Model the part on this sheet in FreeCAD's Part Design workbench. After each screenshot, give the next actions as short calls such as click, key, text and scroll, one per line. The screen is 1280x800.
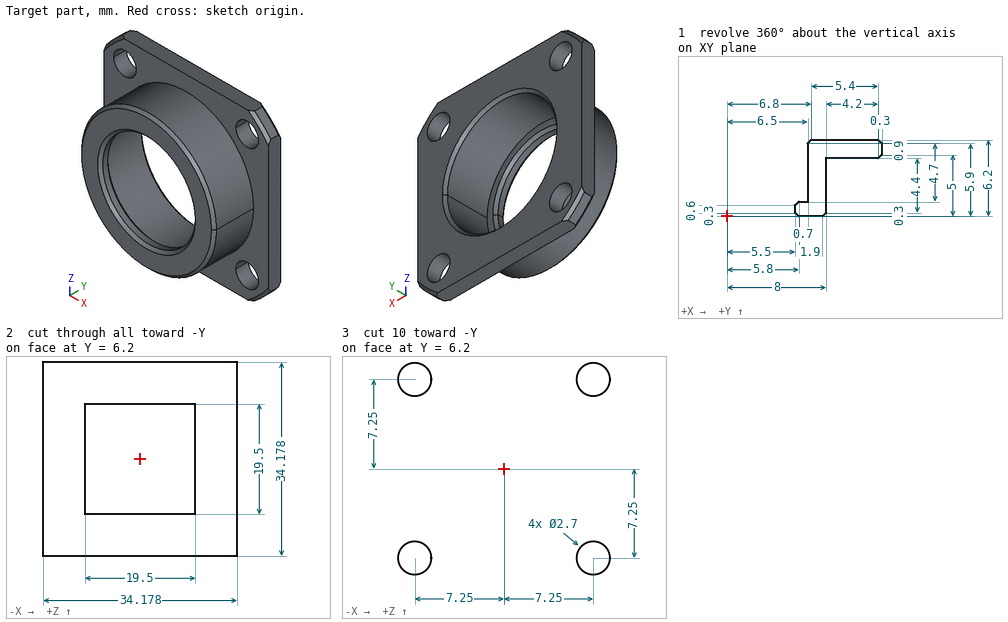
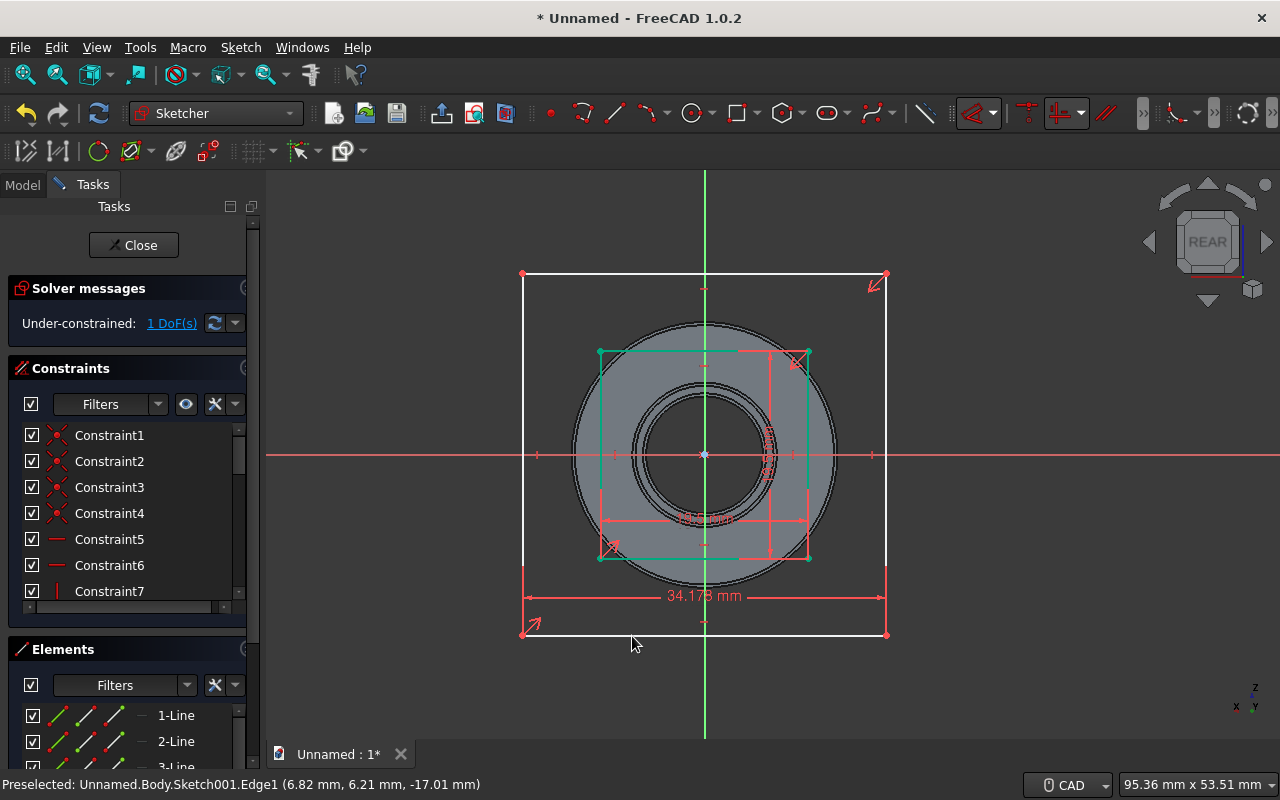
click(886, 527)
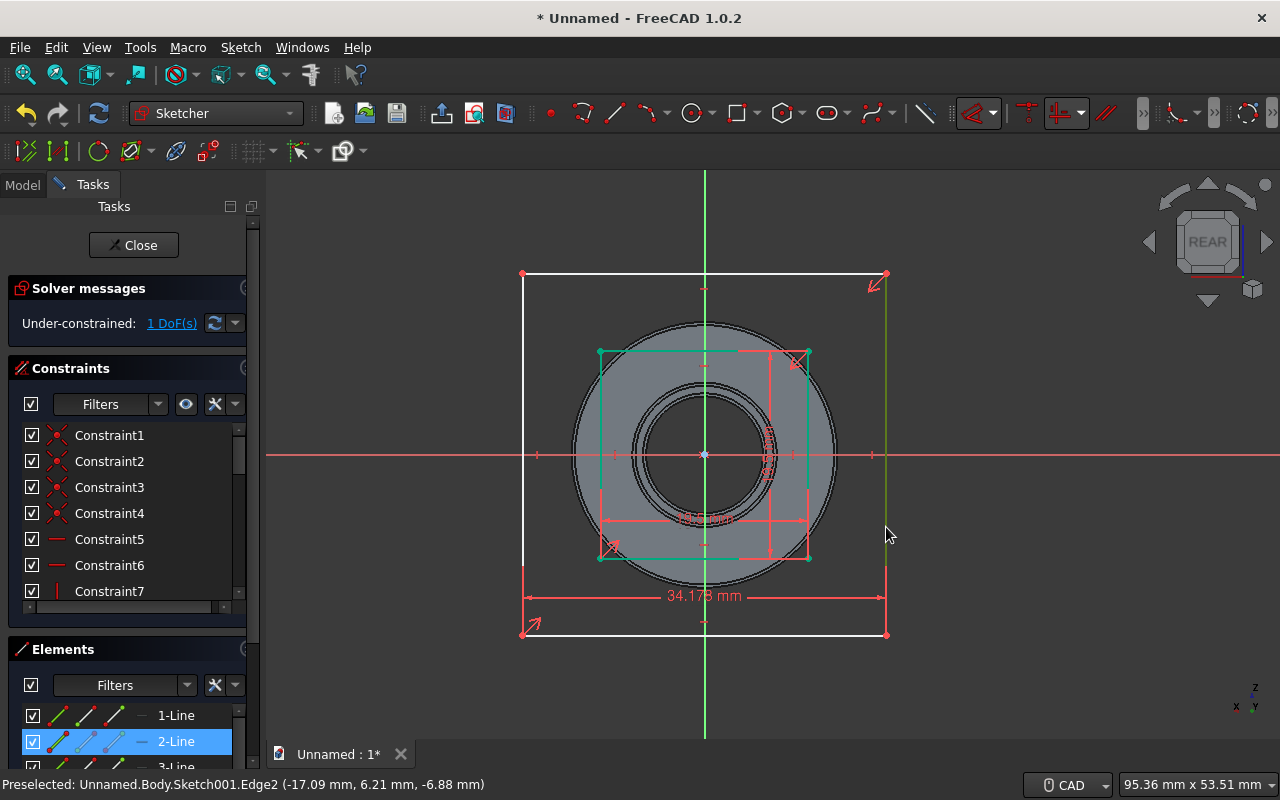
click(996, 114)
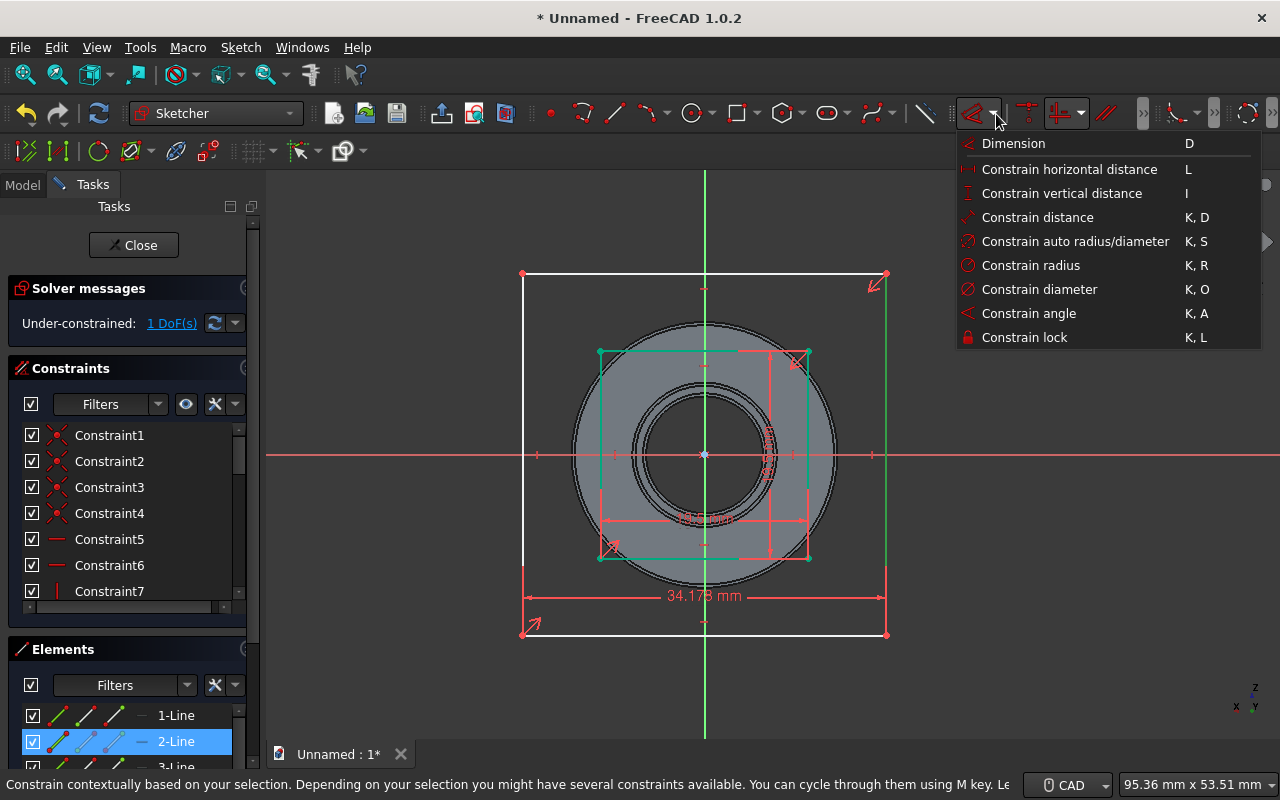
click(1109, 193)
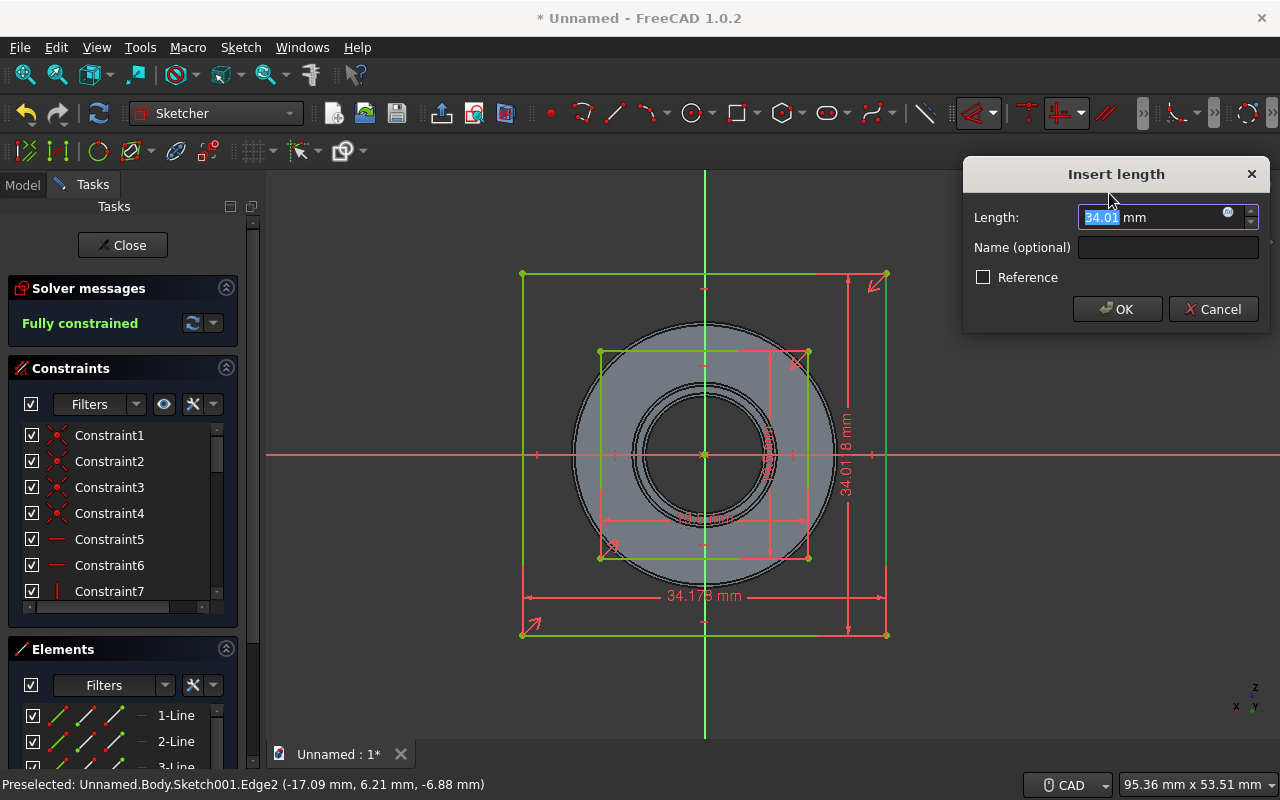
text(34.178)
key(Return)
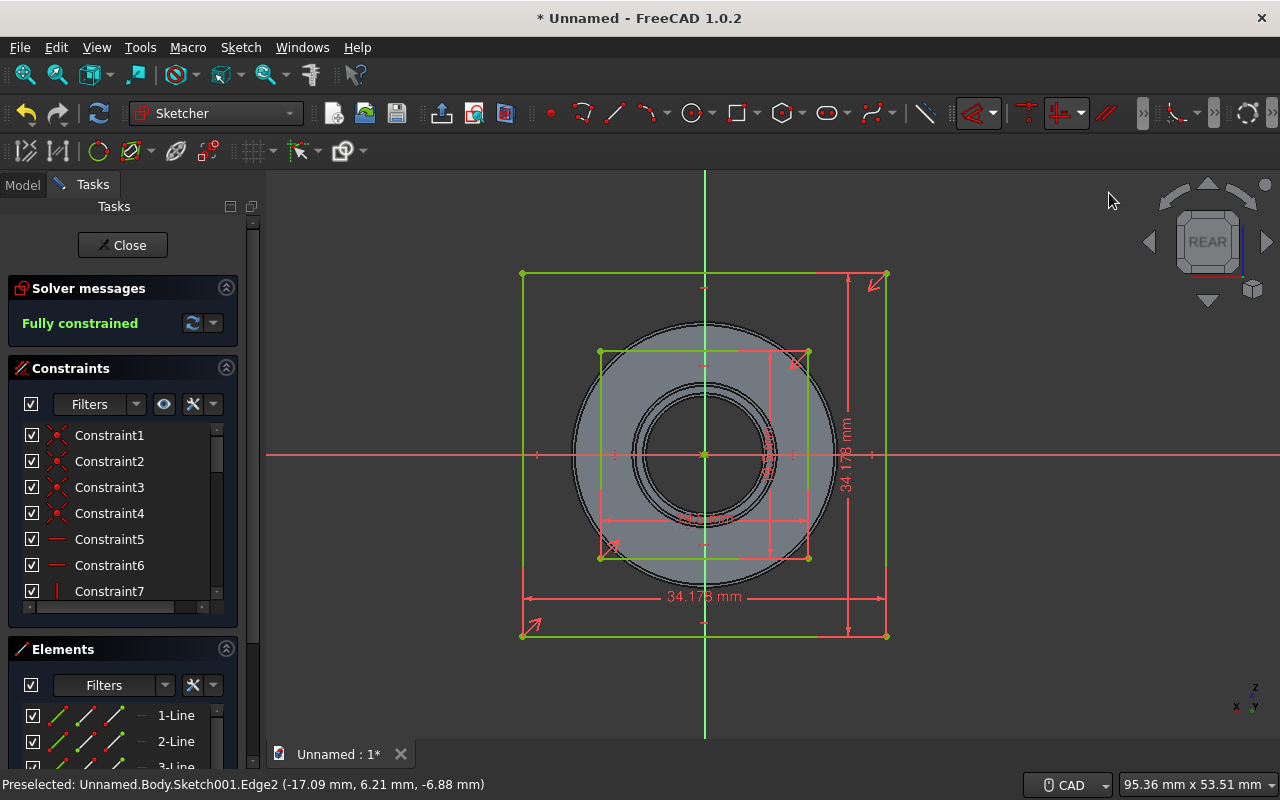
click(123, 245)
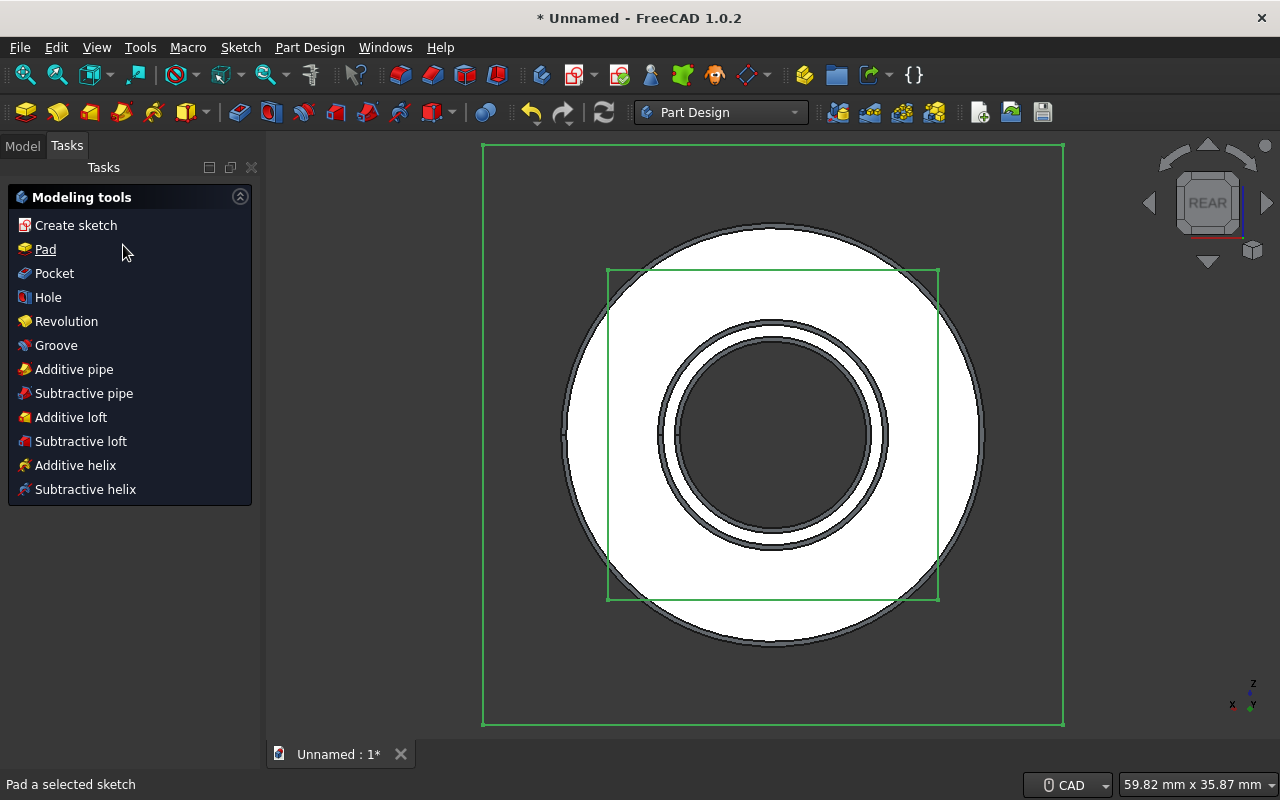
click(240, 112)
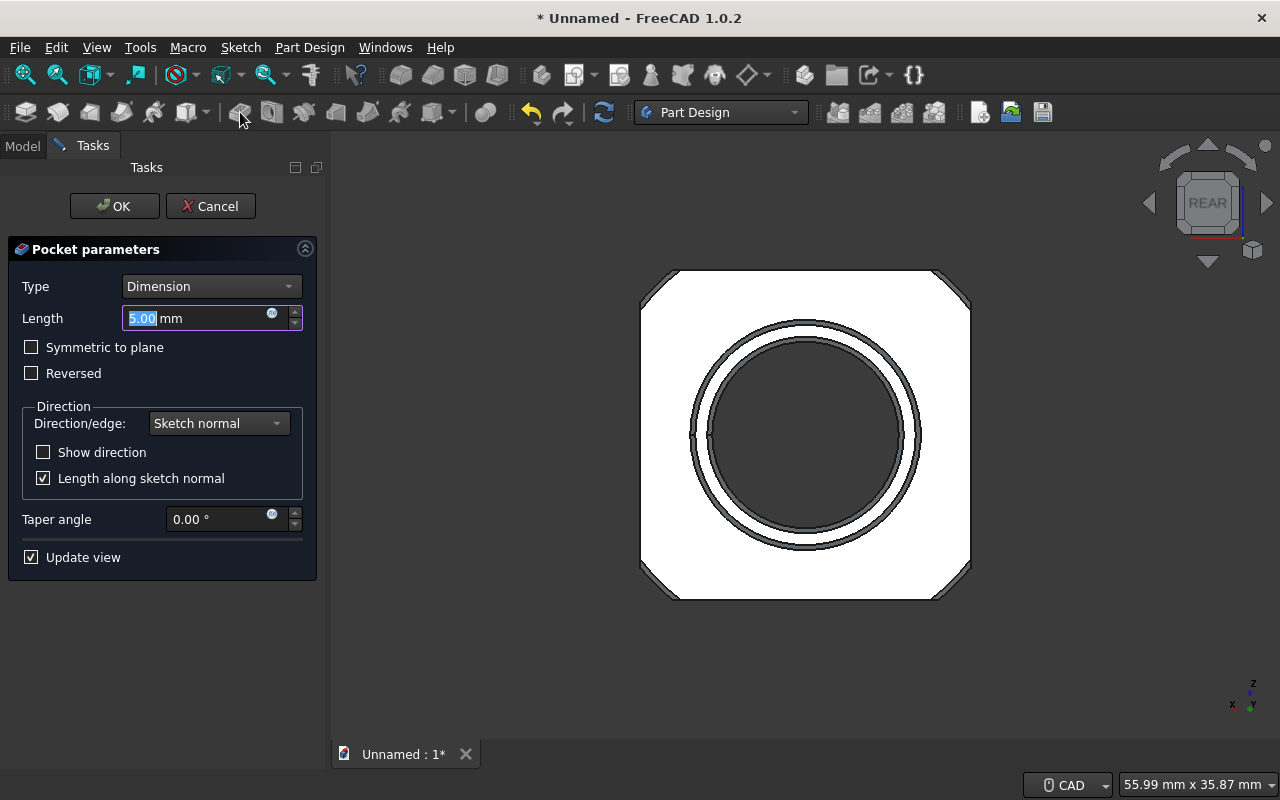
click(212, 286)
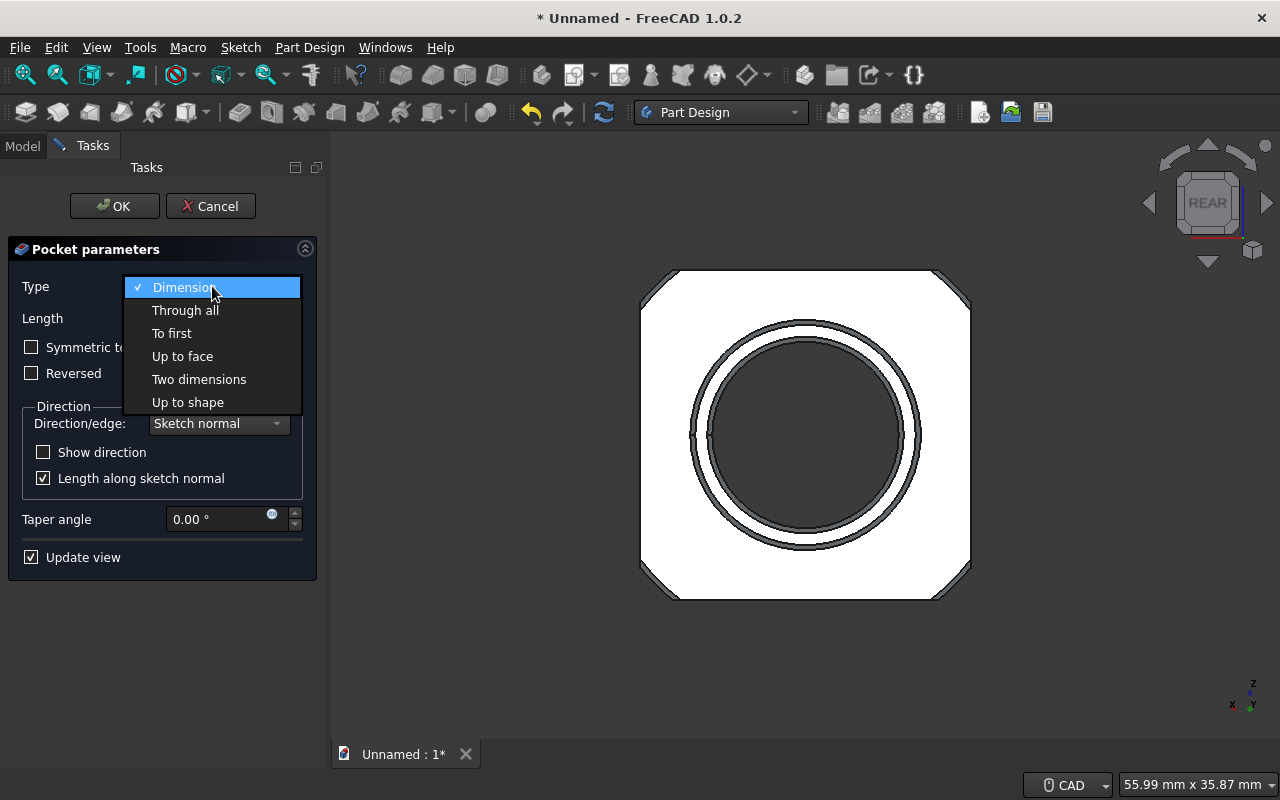
click(212, 310)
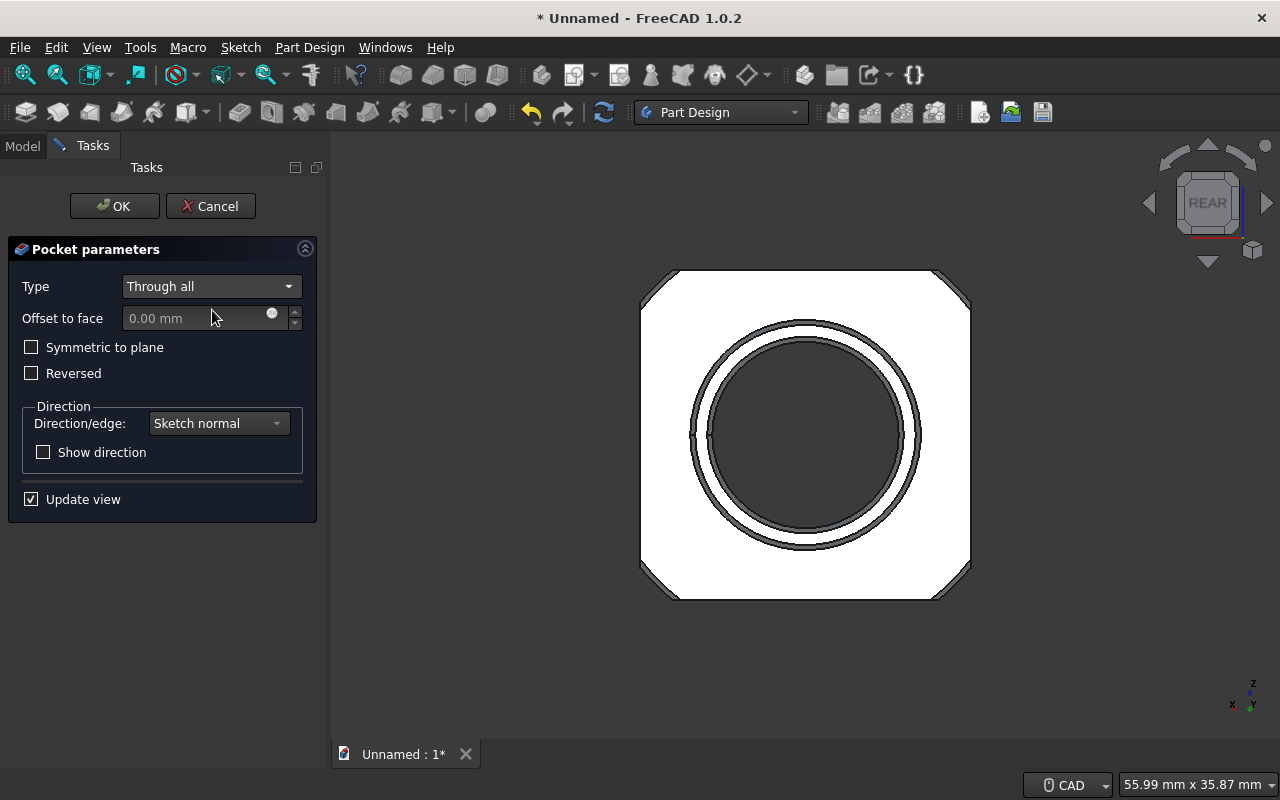
click(115, 206)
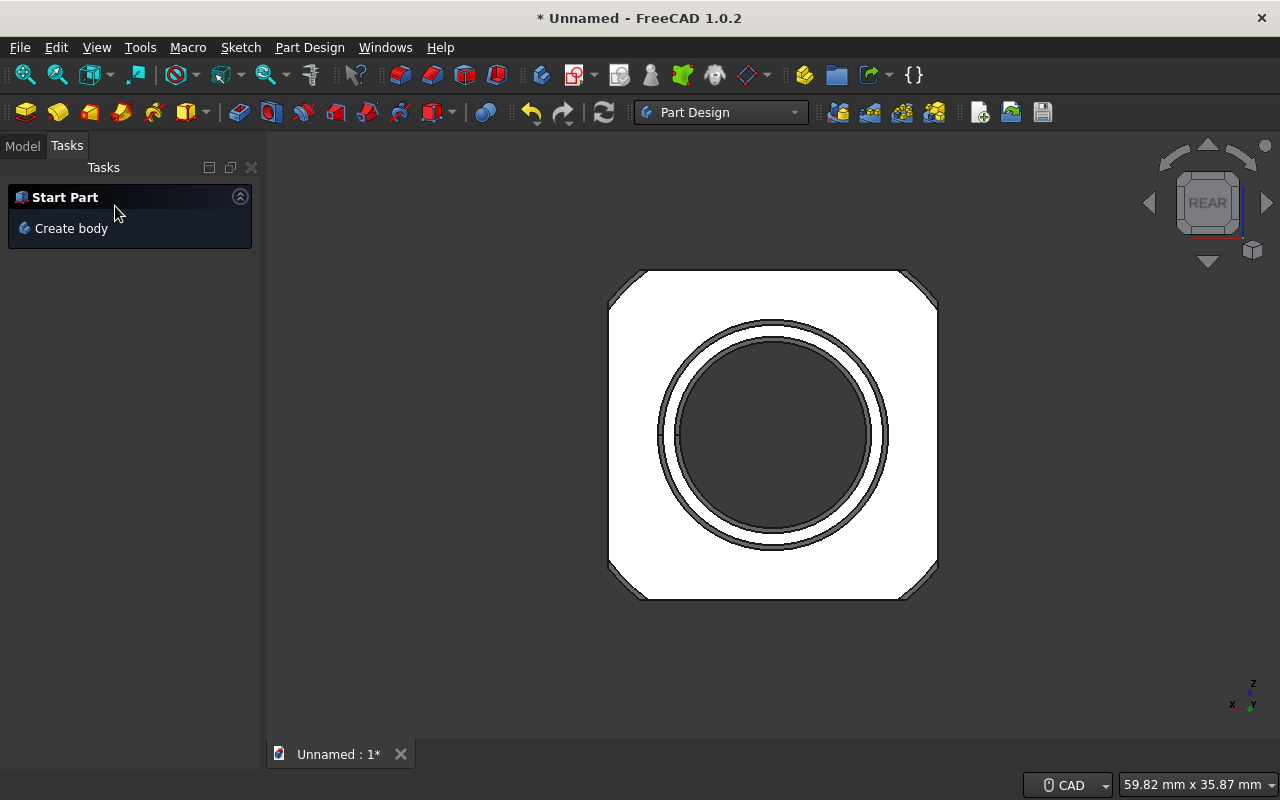
click(631, 340)